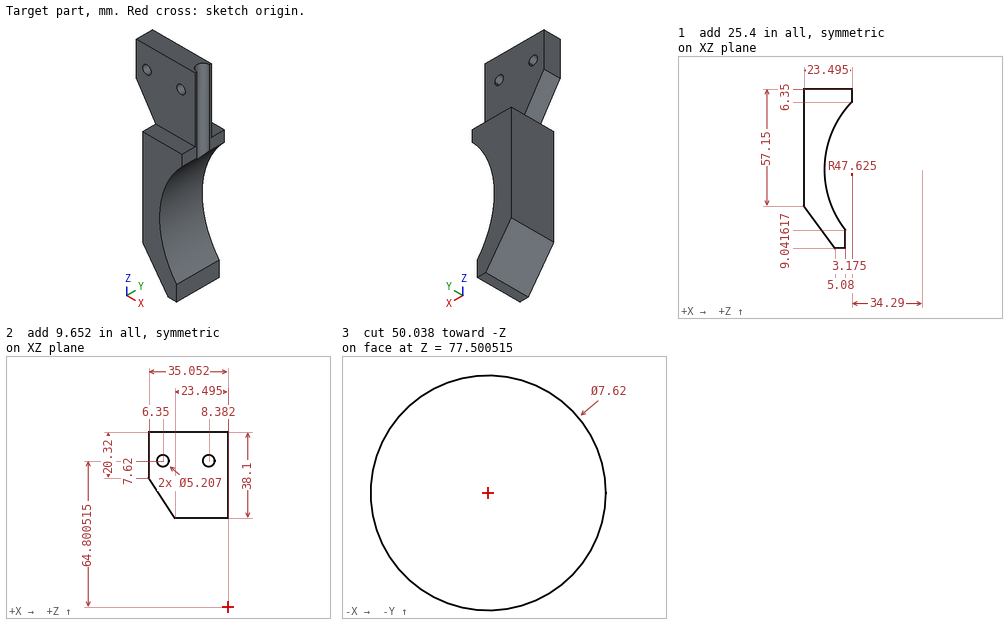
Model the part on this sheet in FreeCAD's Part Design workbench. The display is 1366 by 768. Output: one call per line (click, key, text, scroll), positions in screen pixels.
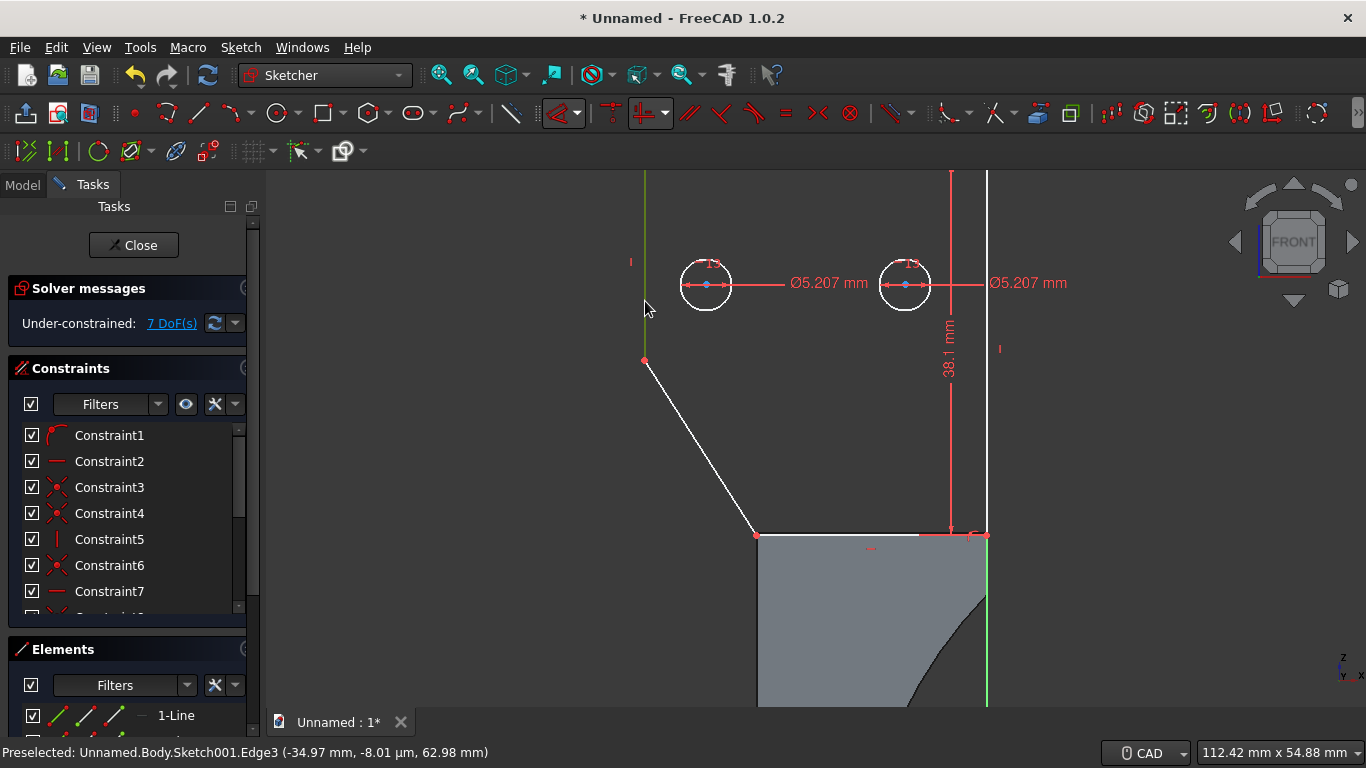
key(i)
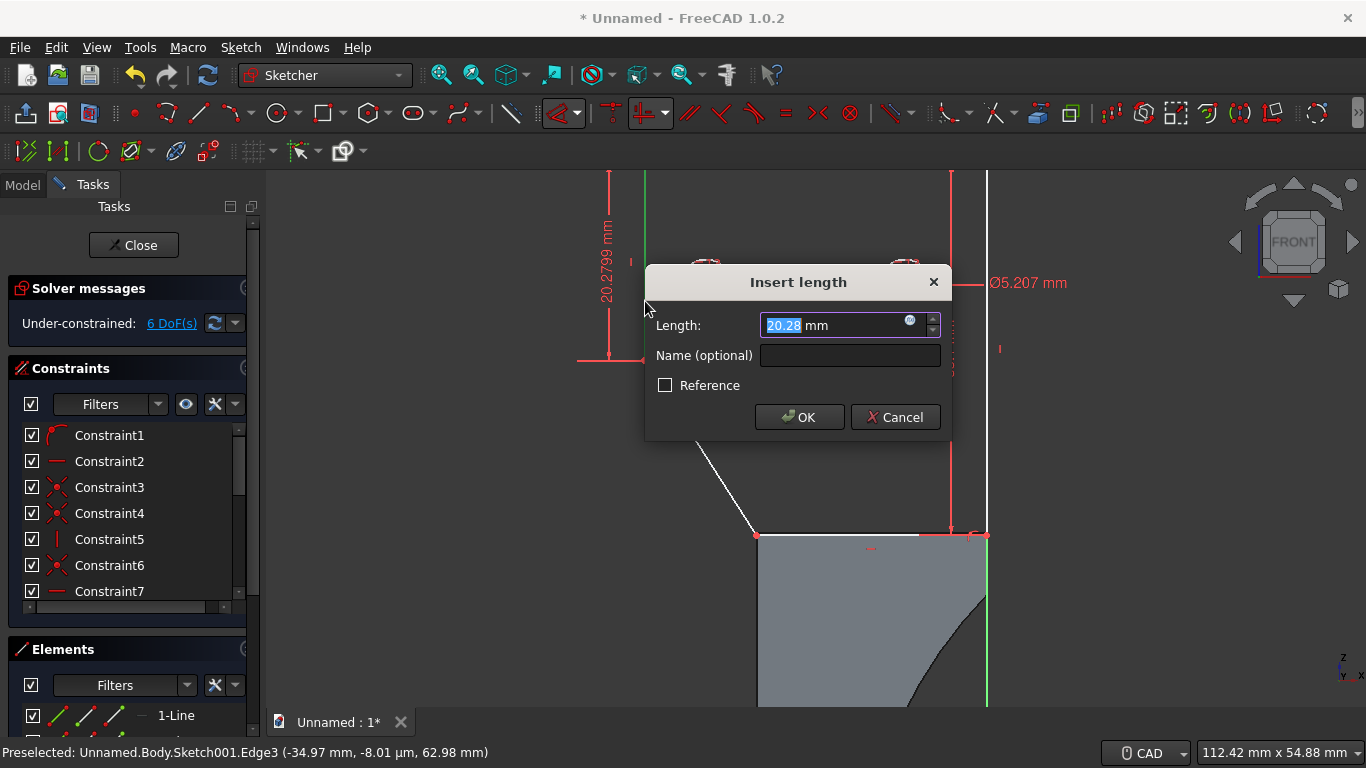
text(20.32)
key(Return)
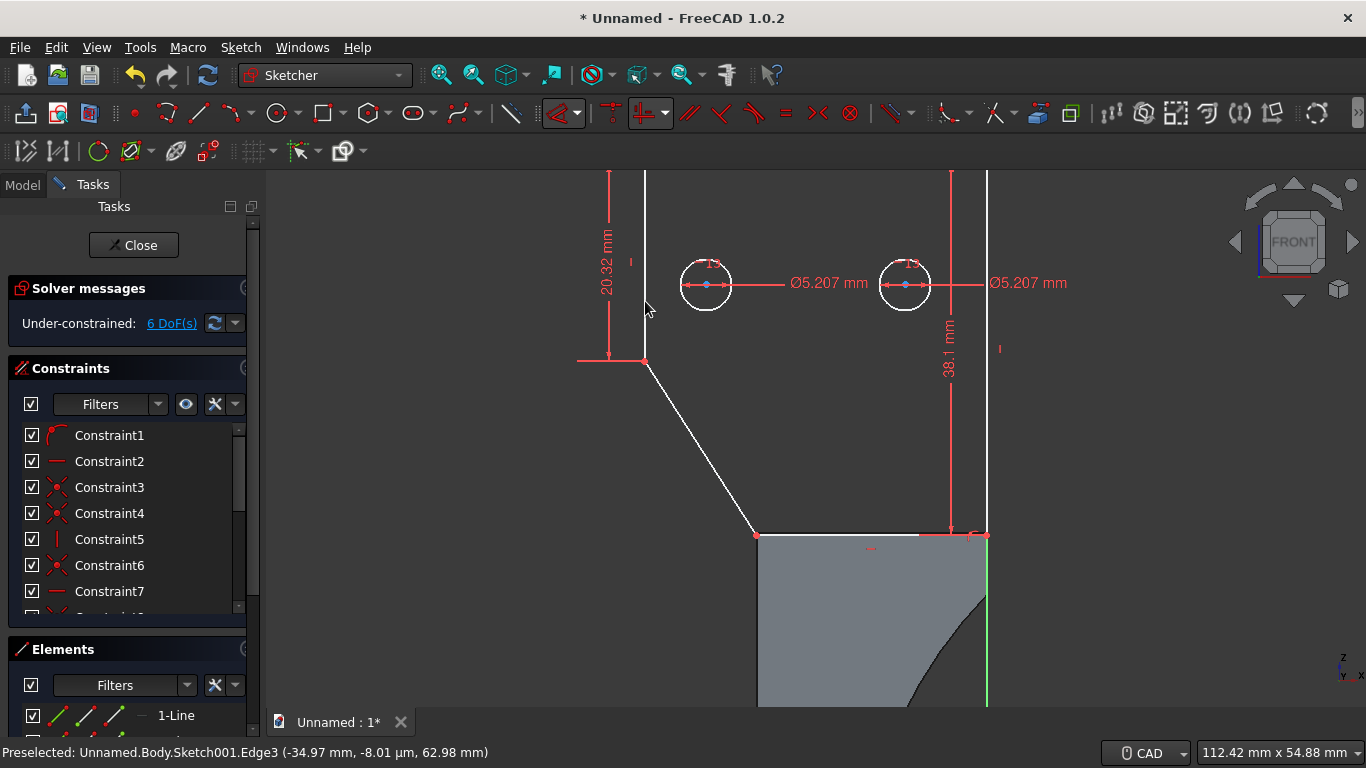
click(905, 285)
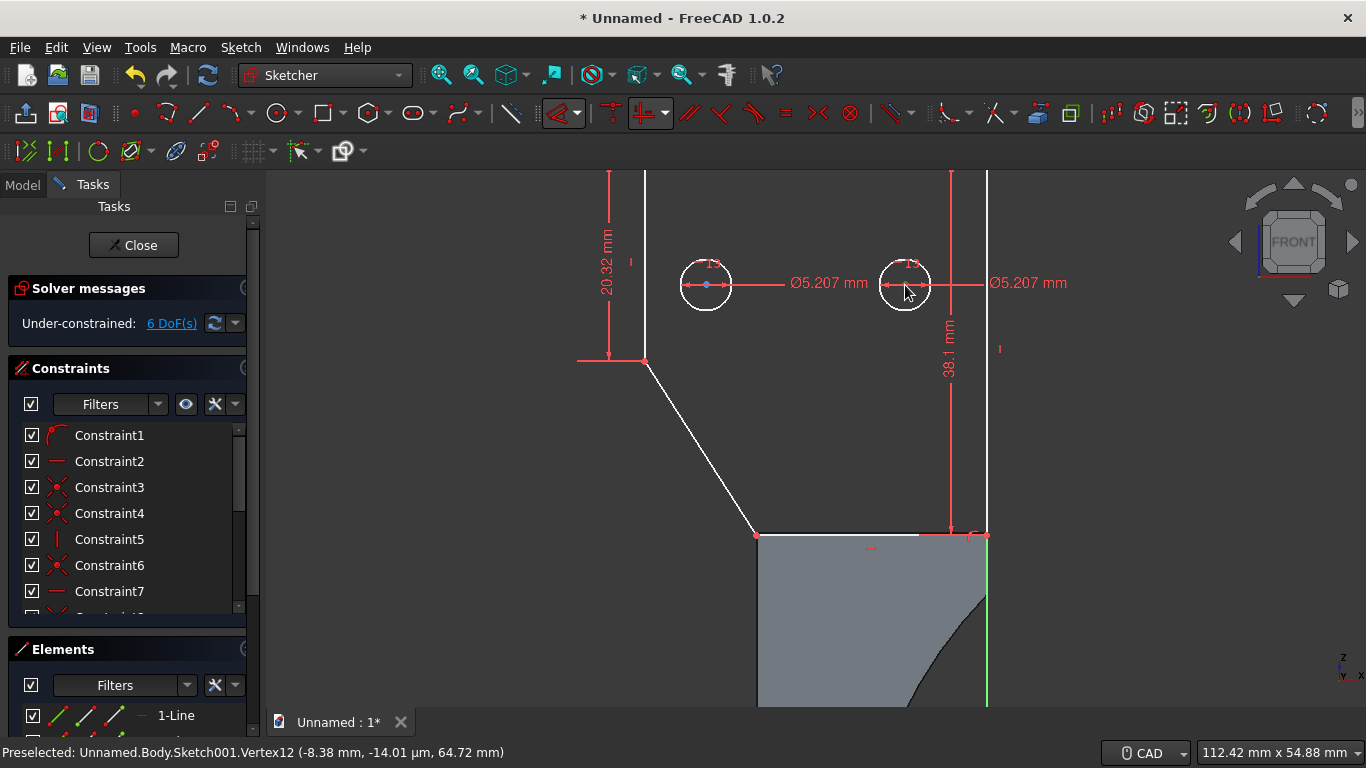
click(580, 114)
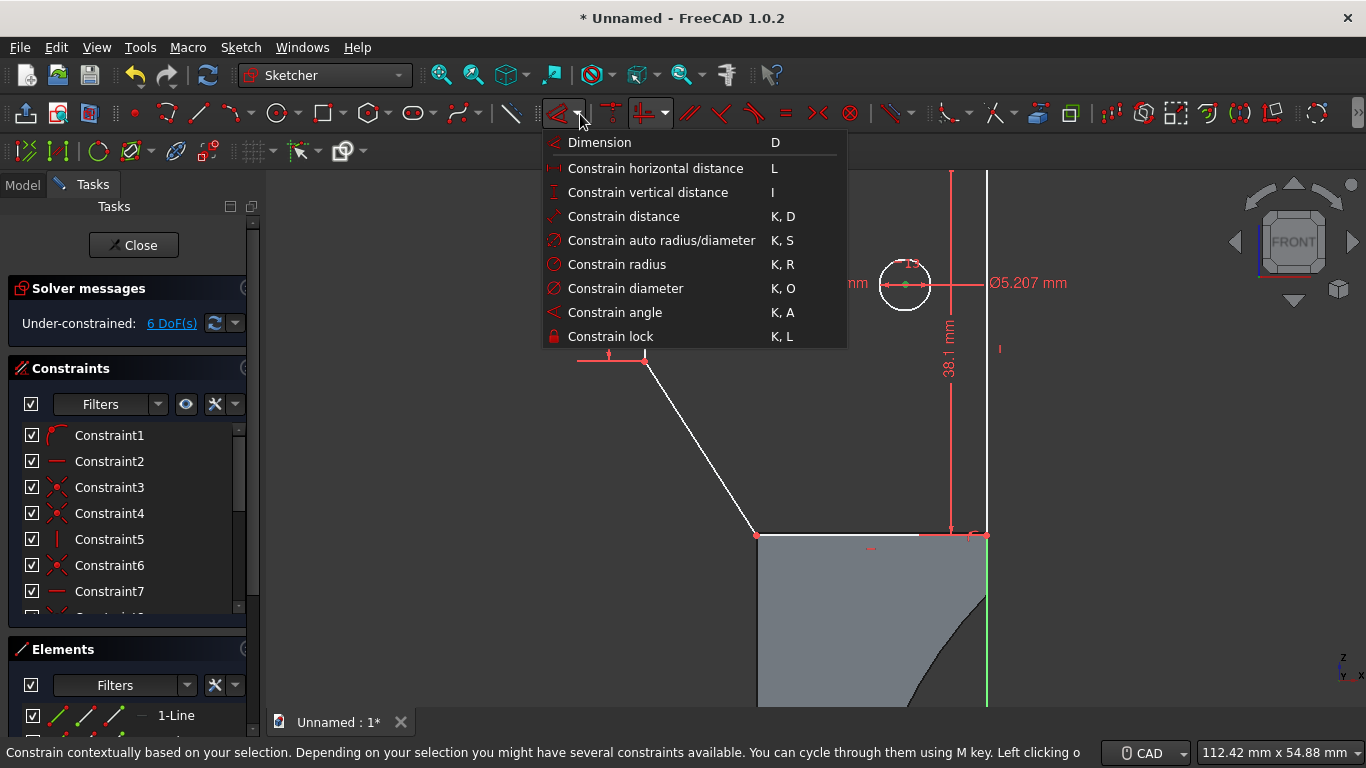
click(695, 168)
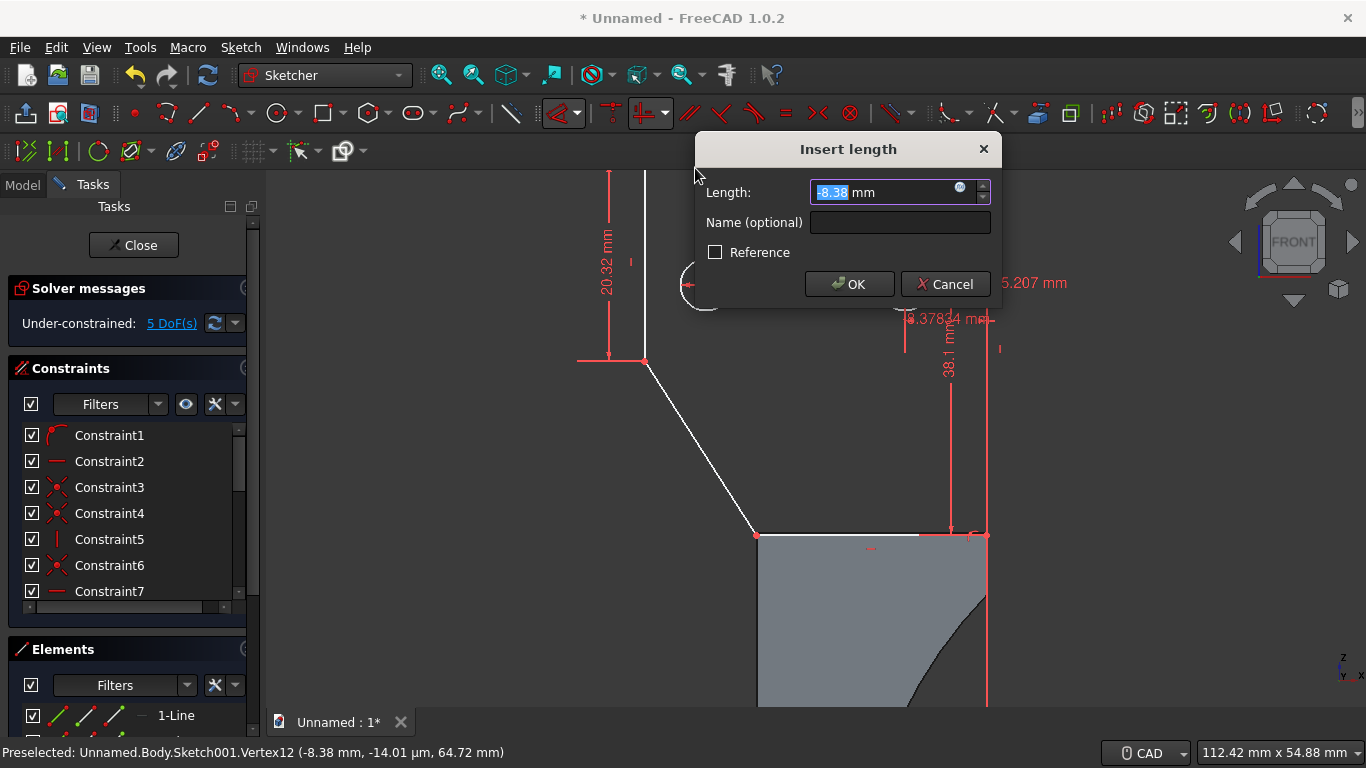
text(-8.382)
key(Return)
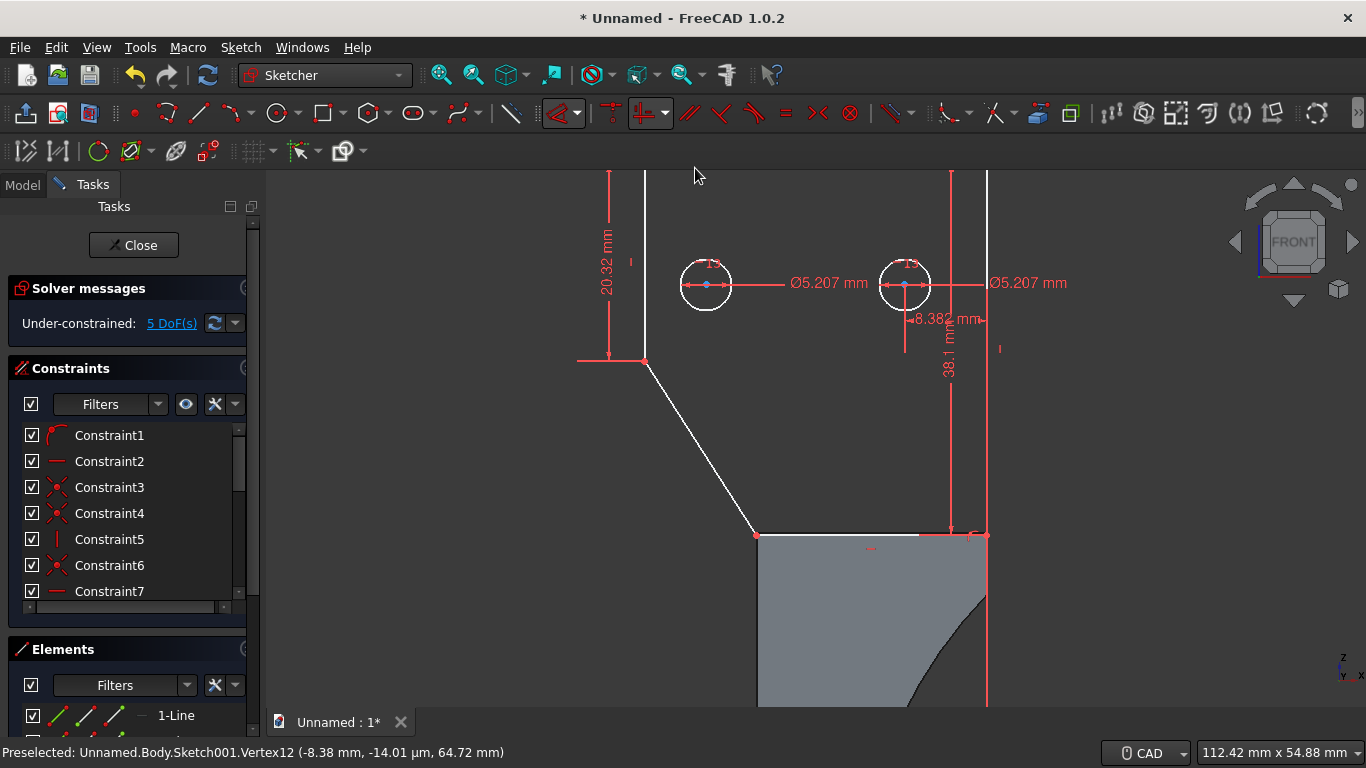
click(645, 361)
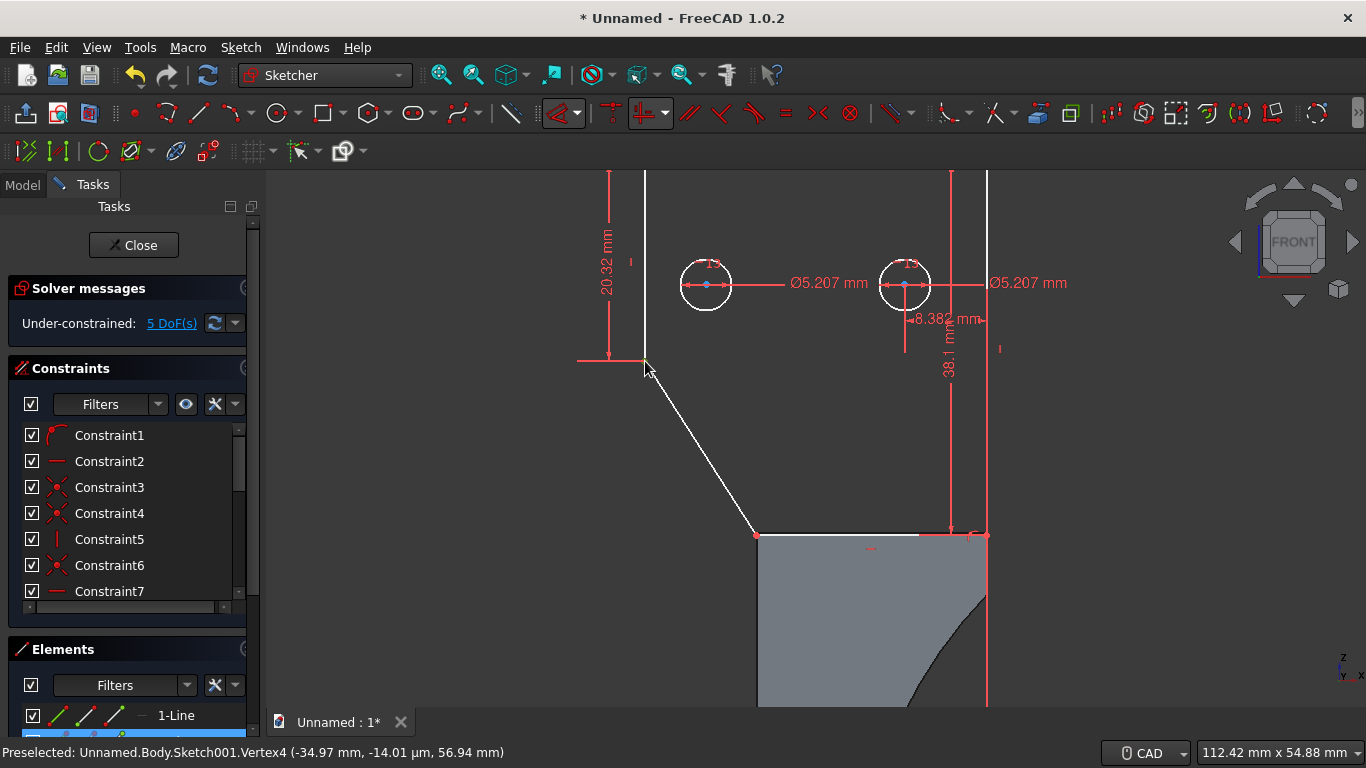
click(706, 285)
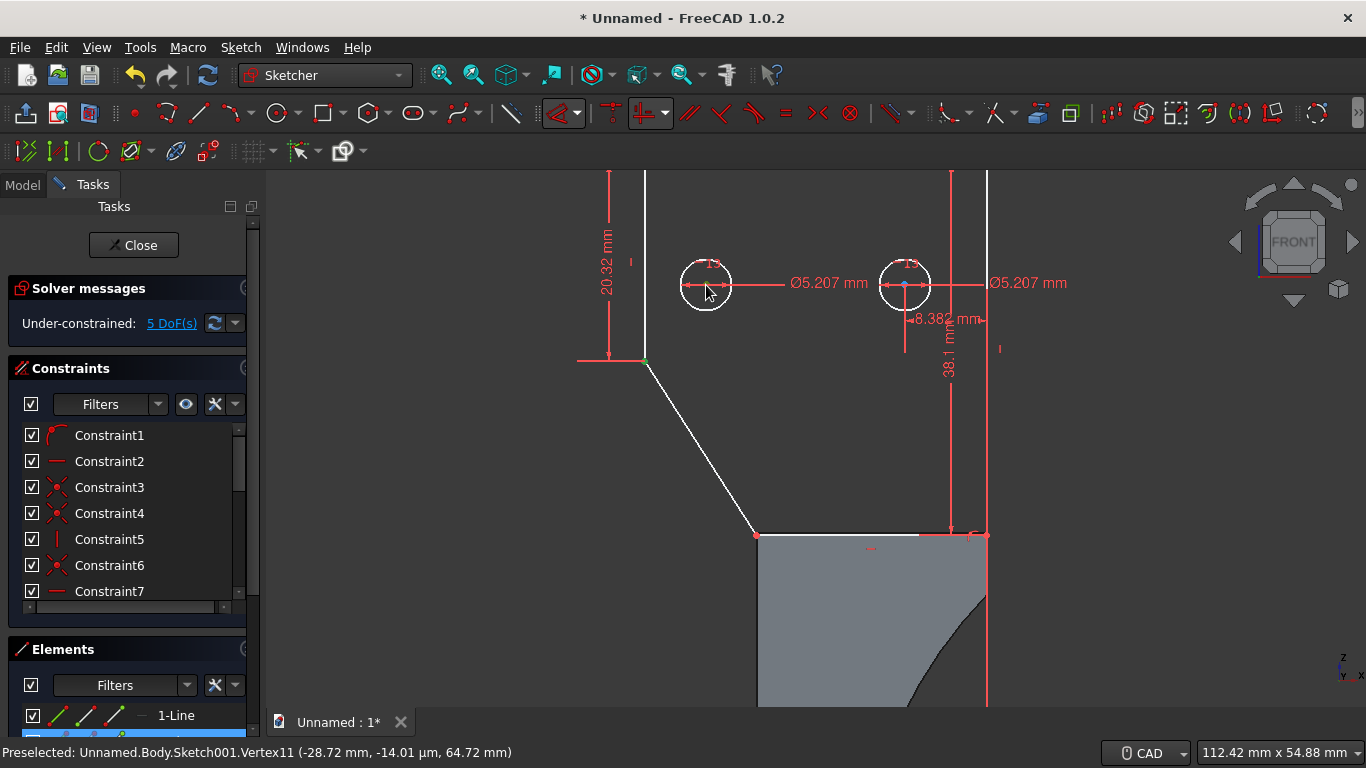
click(580, 114)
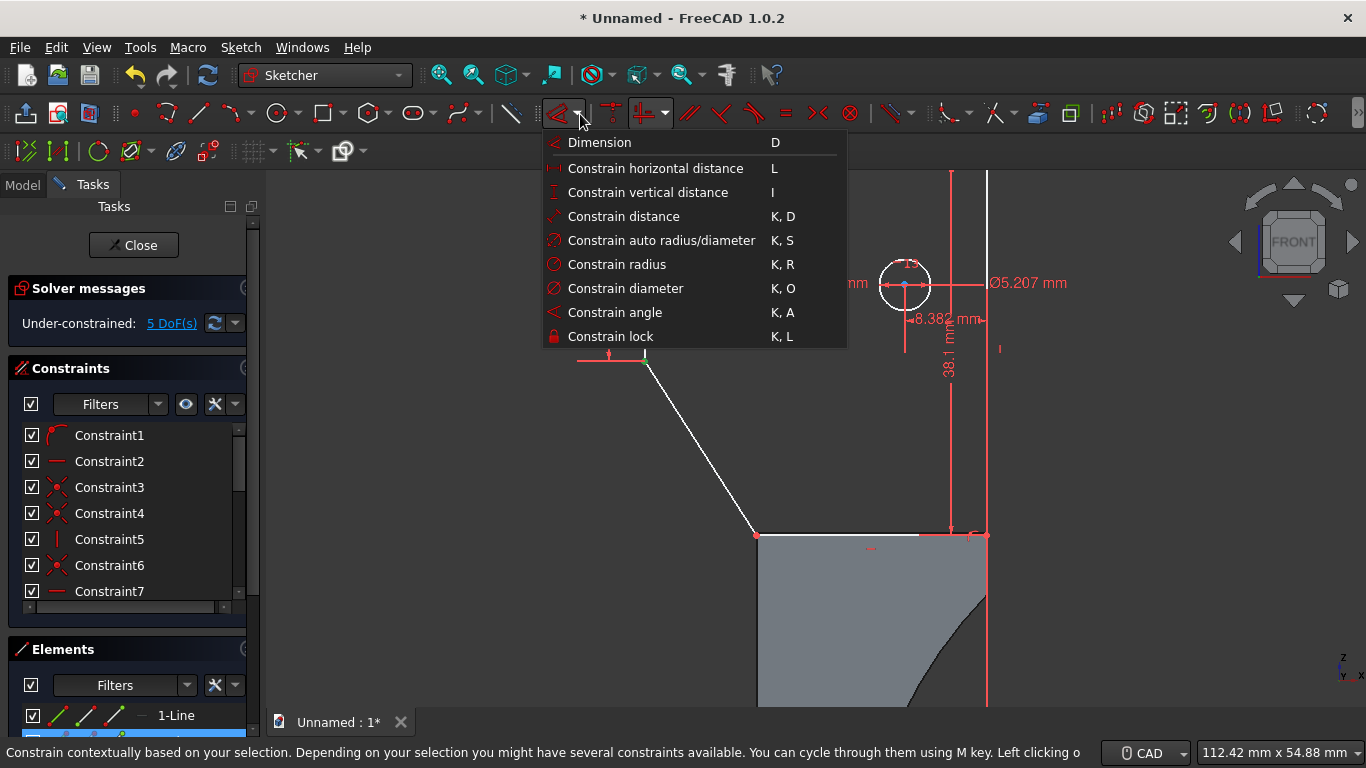
click(695, 168)